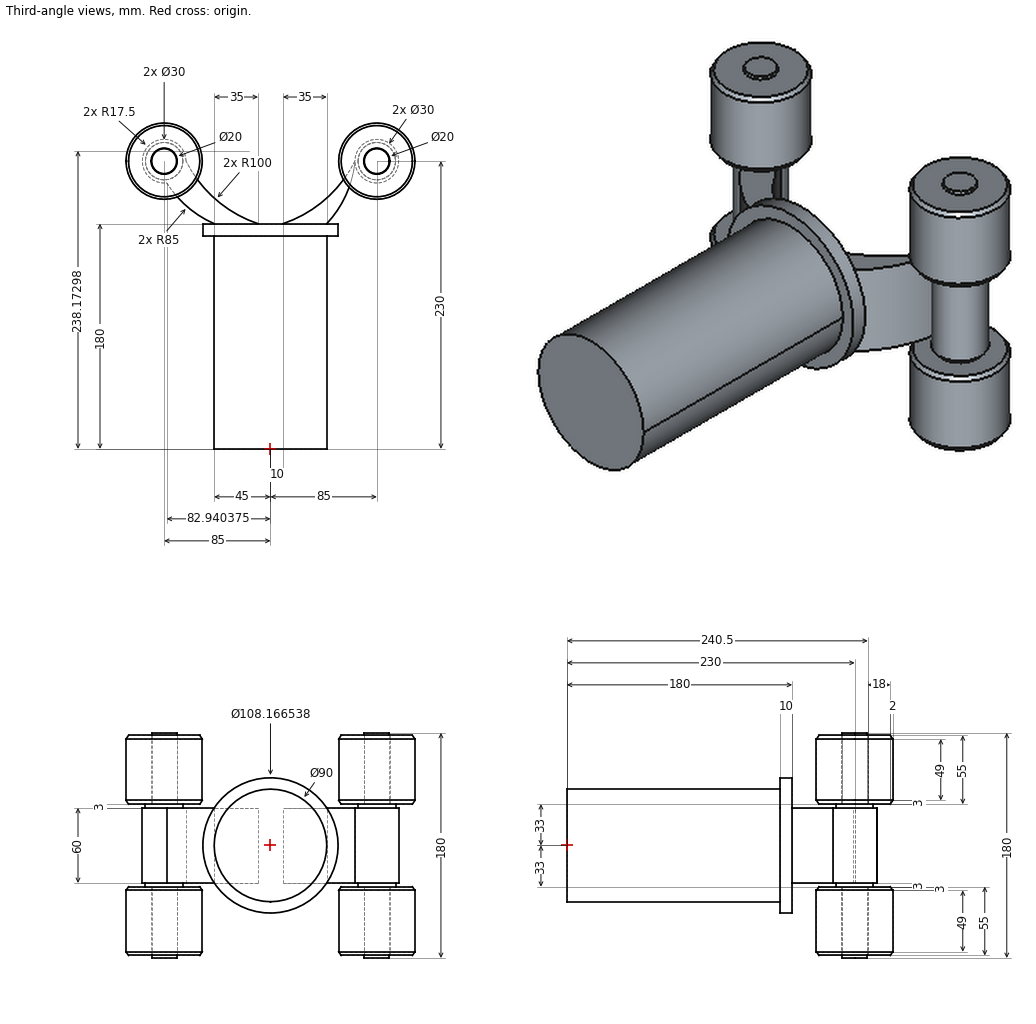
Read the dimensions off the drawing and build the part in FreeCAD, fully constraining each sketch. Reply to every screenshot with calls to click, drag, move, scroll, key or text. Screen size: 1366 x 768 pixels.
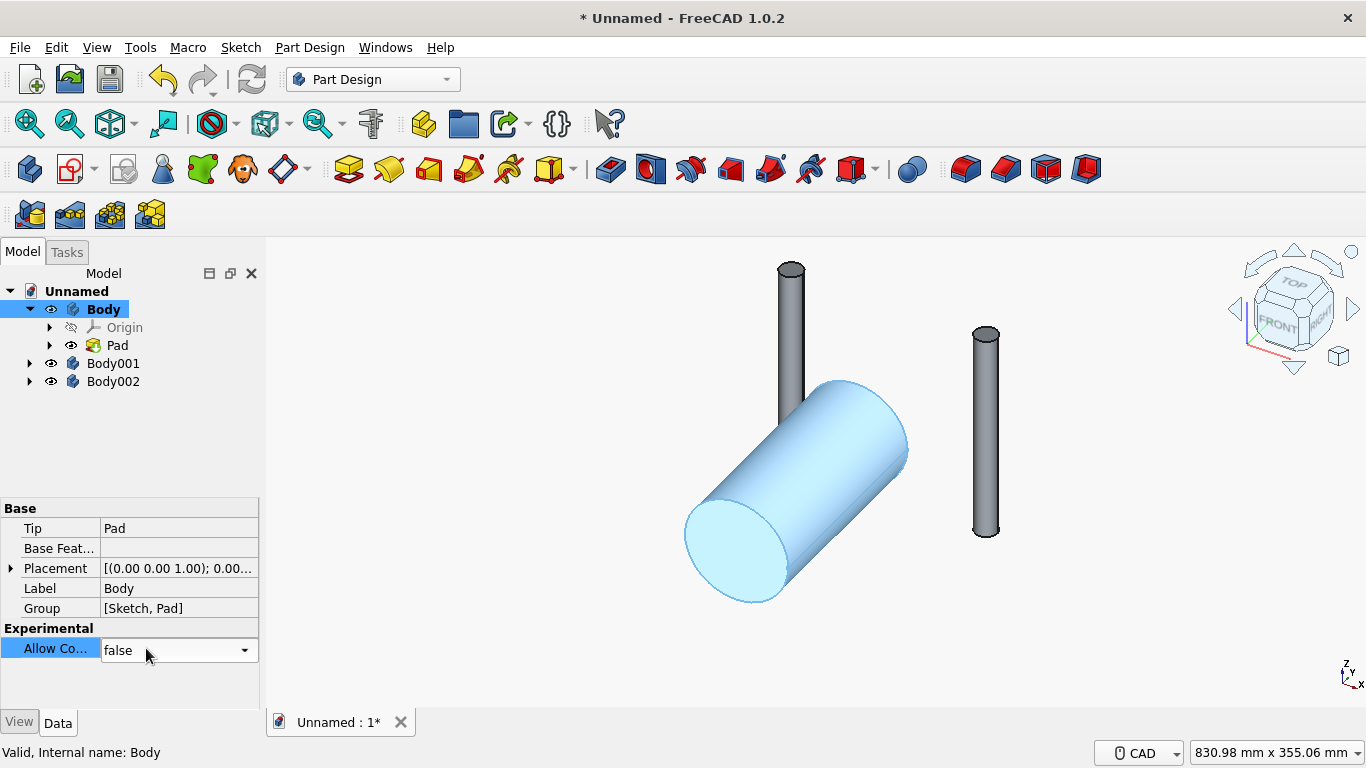
click(146, 648)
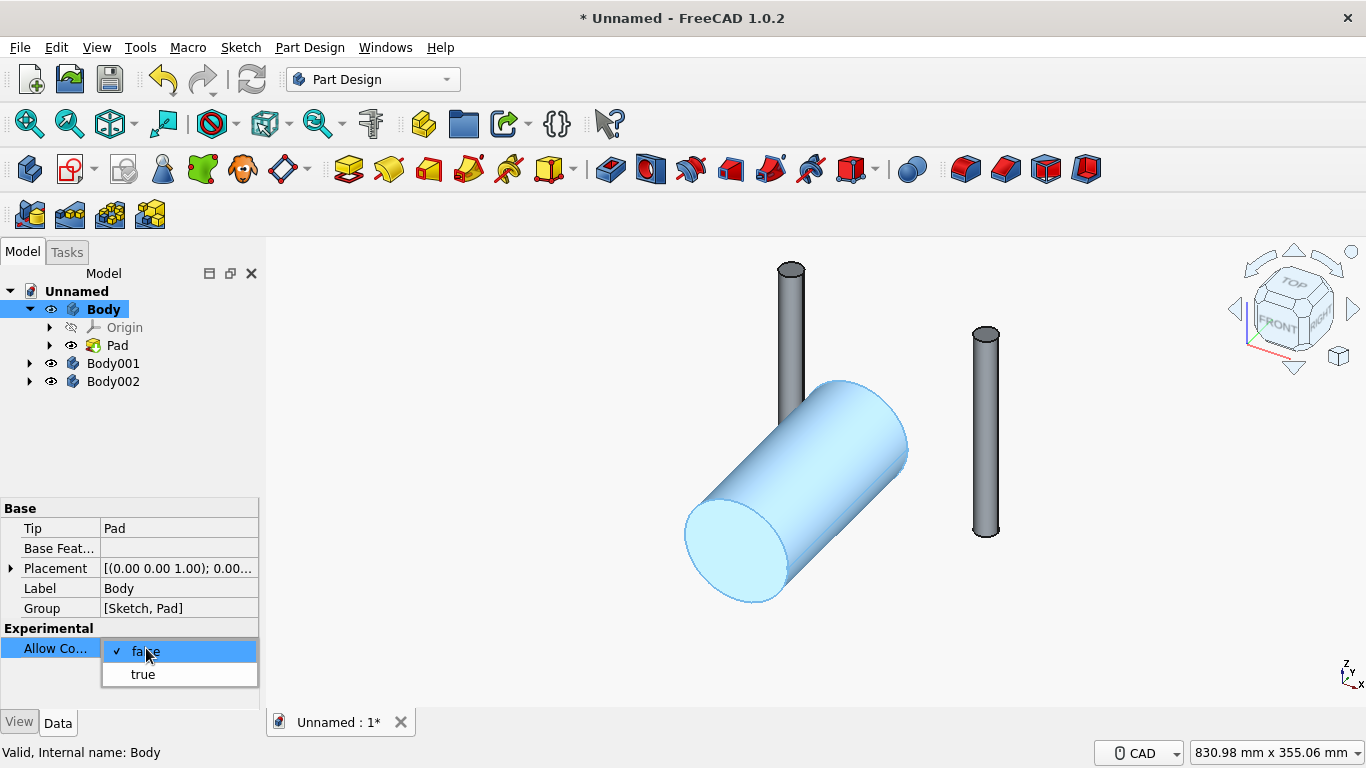
click(179, 674)
key(Return)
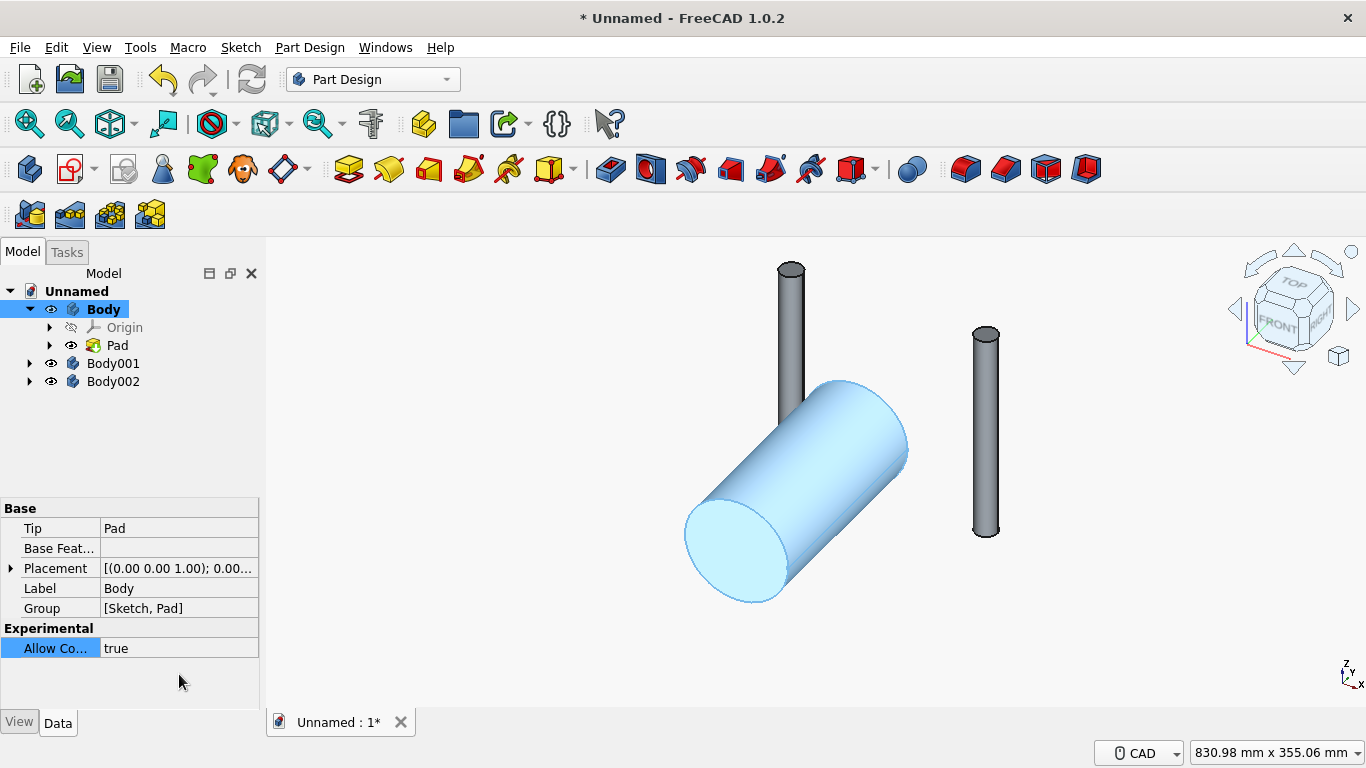
click(96, 363)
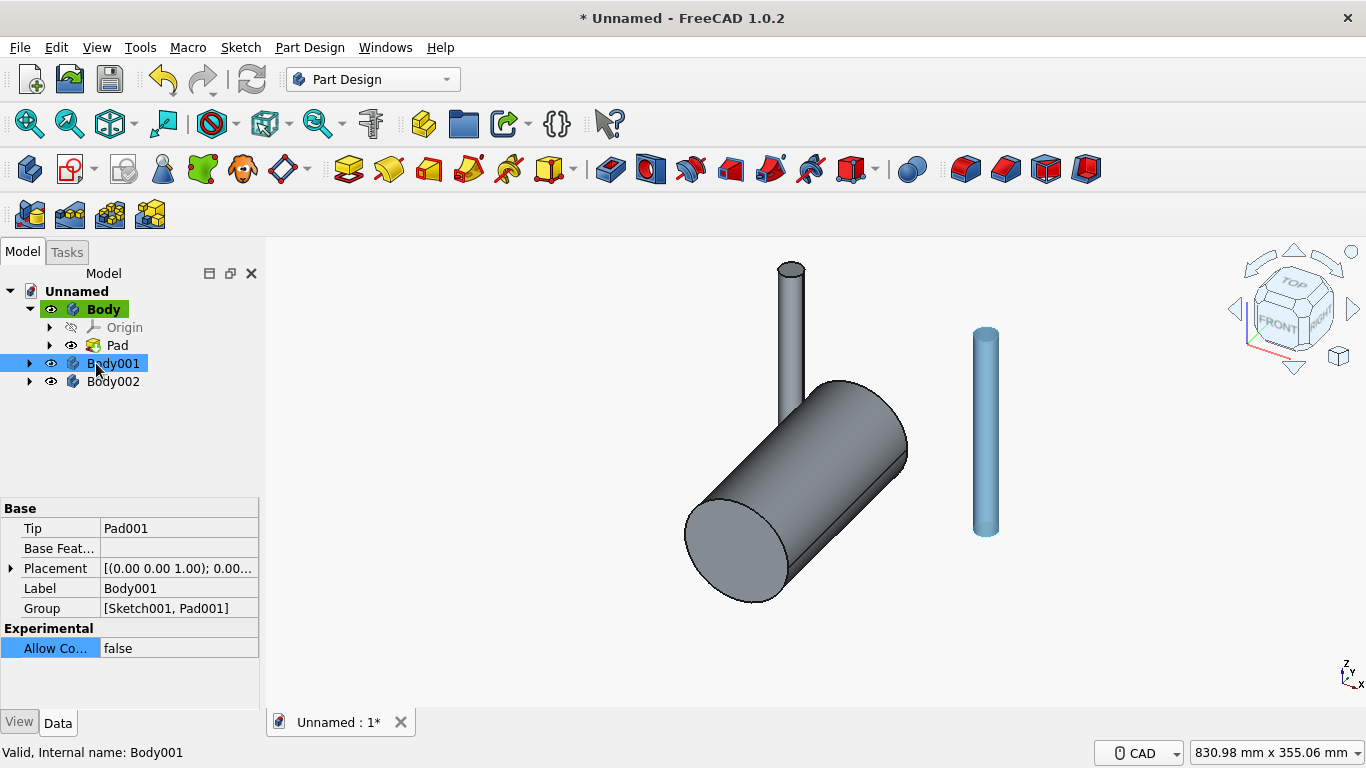
click(914, 170)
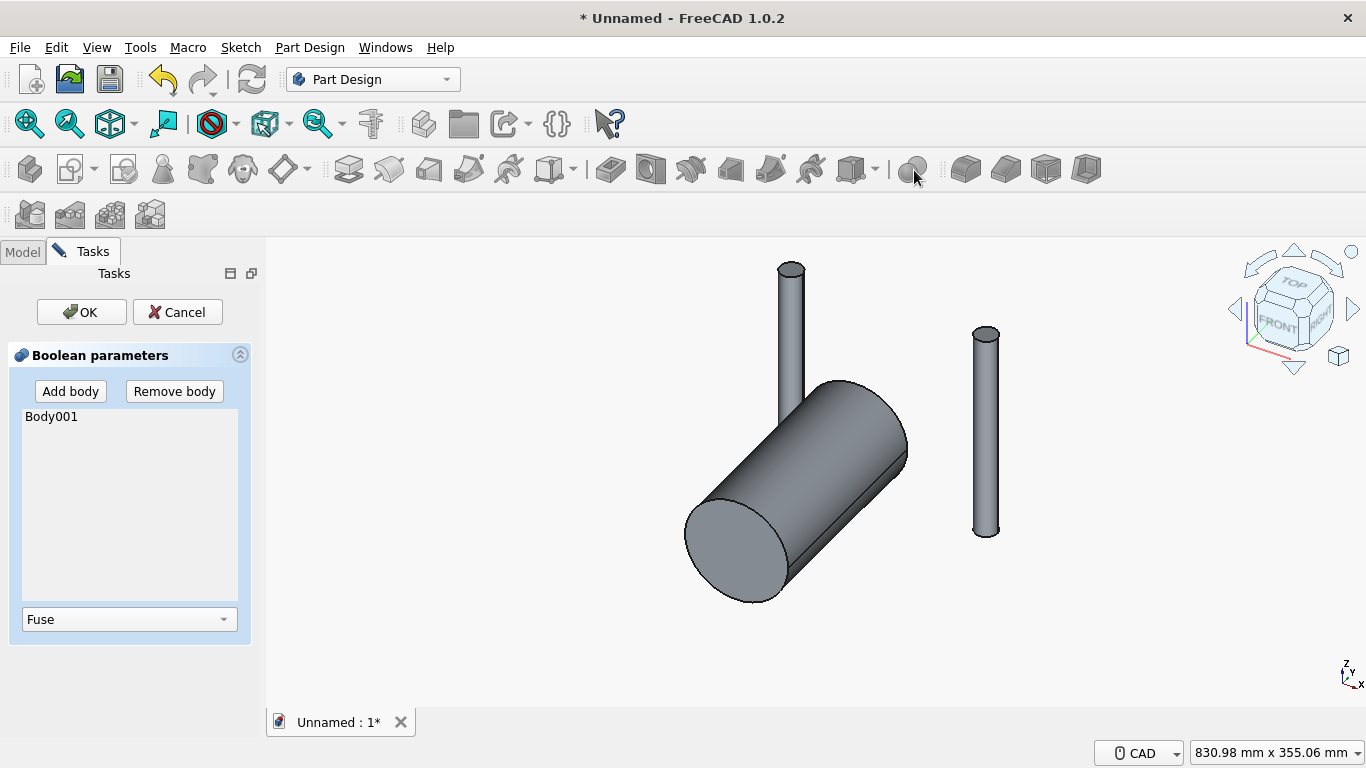
click(82, 312)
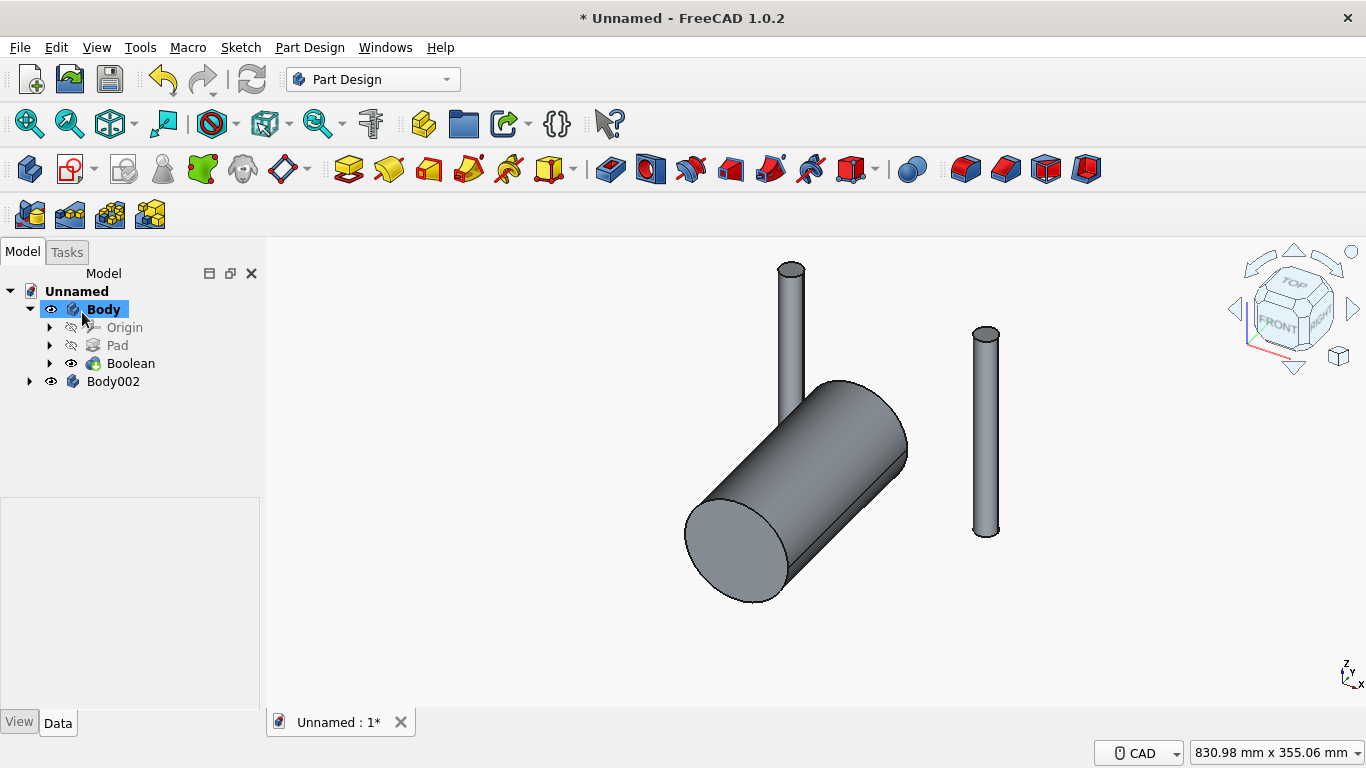
click(96, 381)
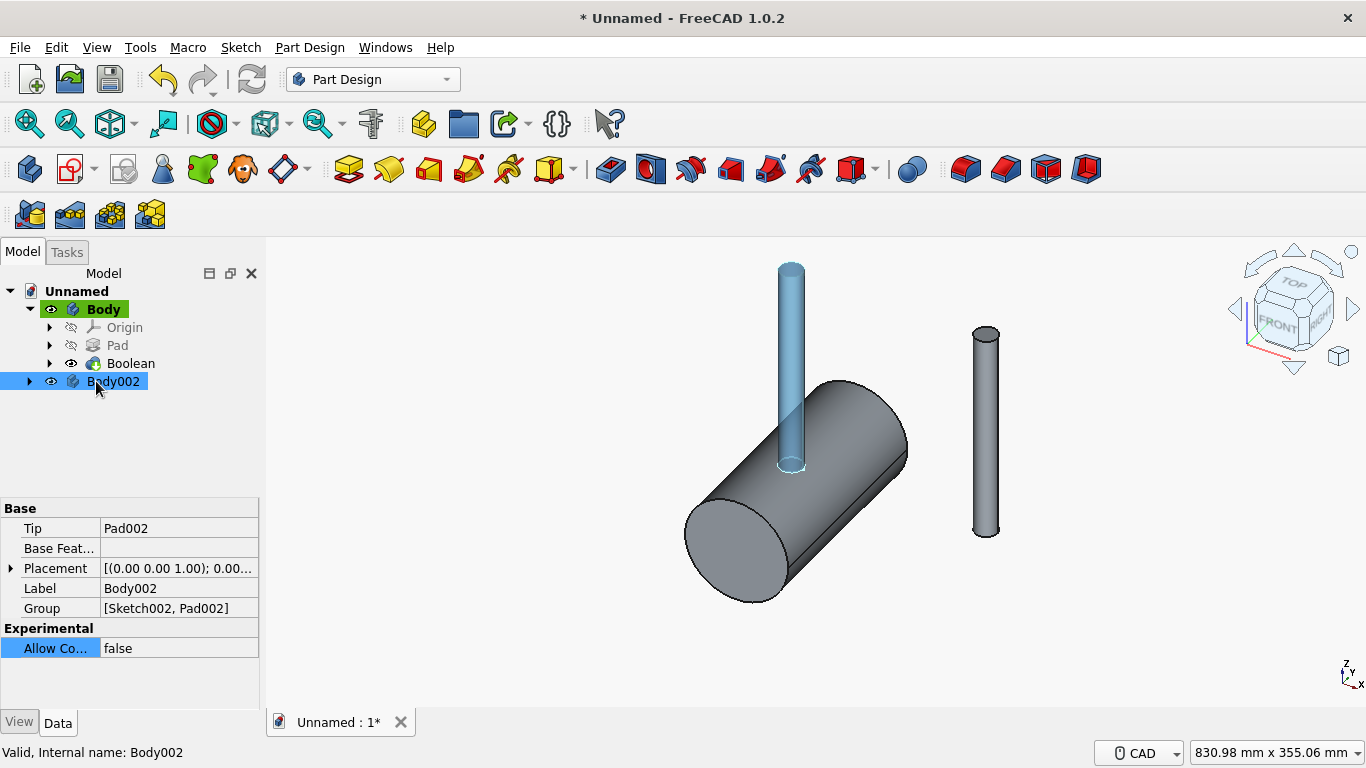
click(914, 170)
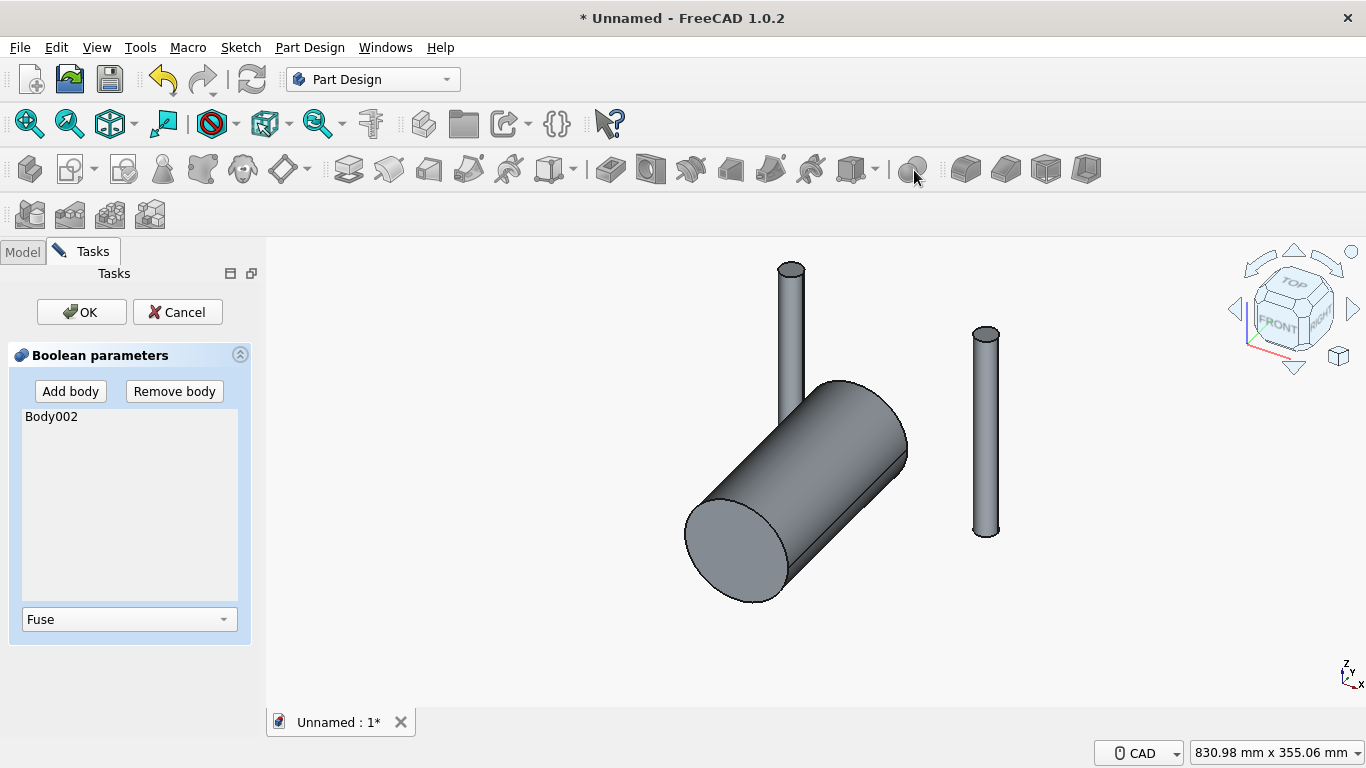
click(82, 312)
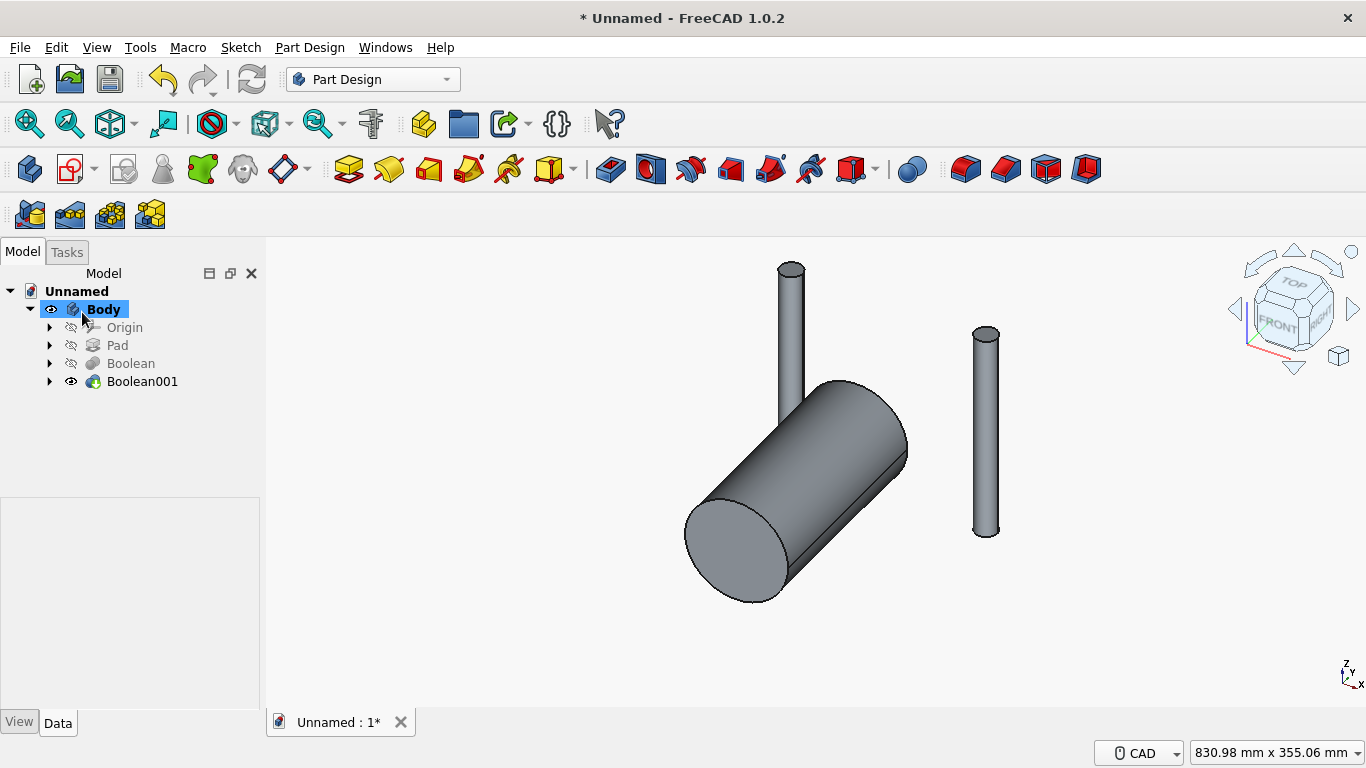
click(70, 170)